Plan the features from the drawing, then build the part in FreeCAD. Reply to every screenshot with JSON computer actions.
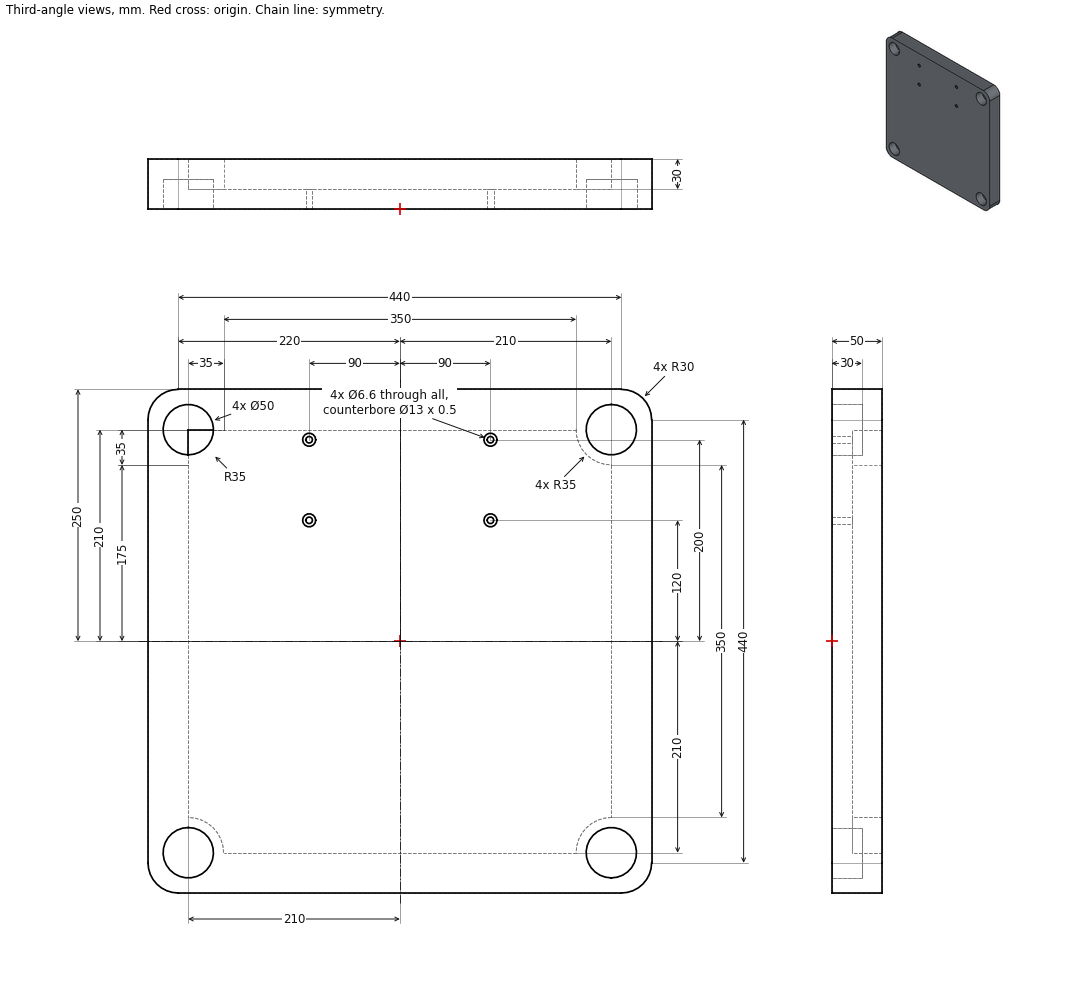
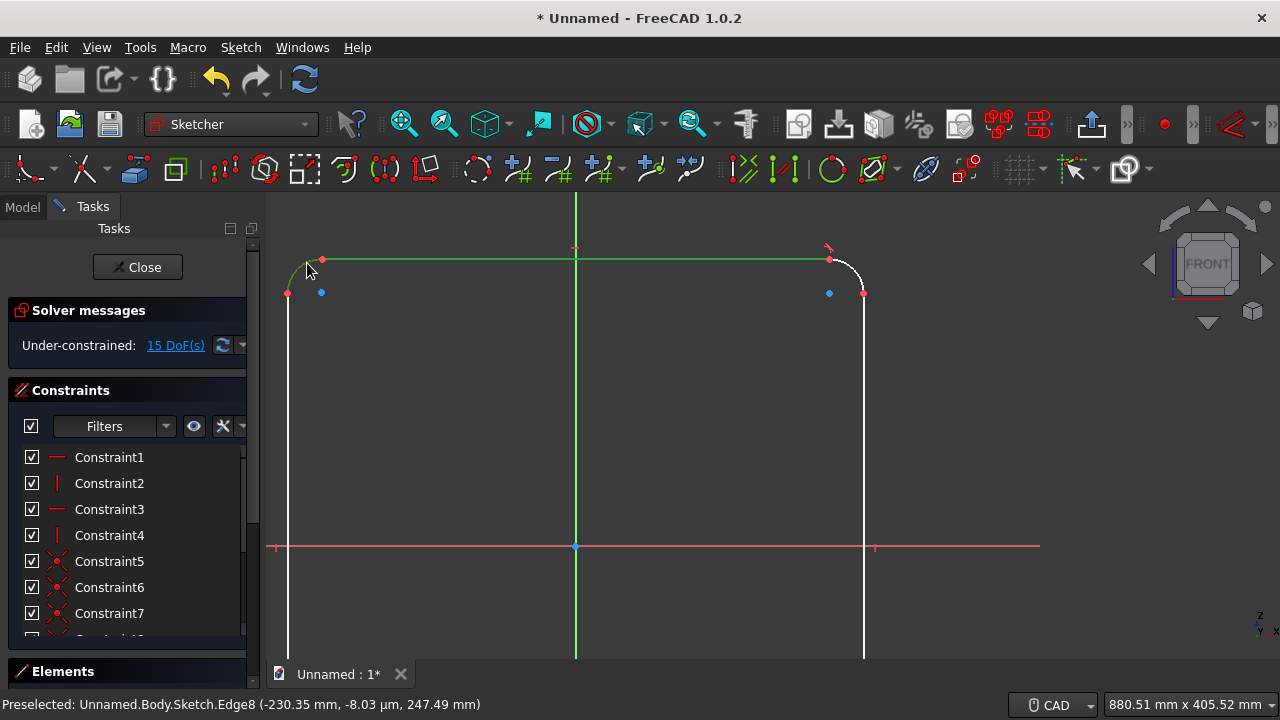
{"action": "key", "text": "t"}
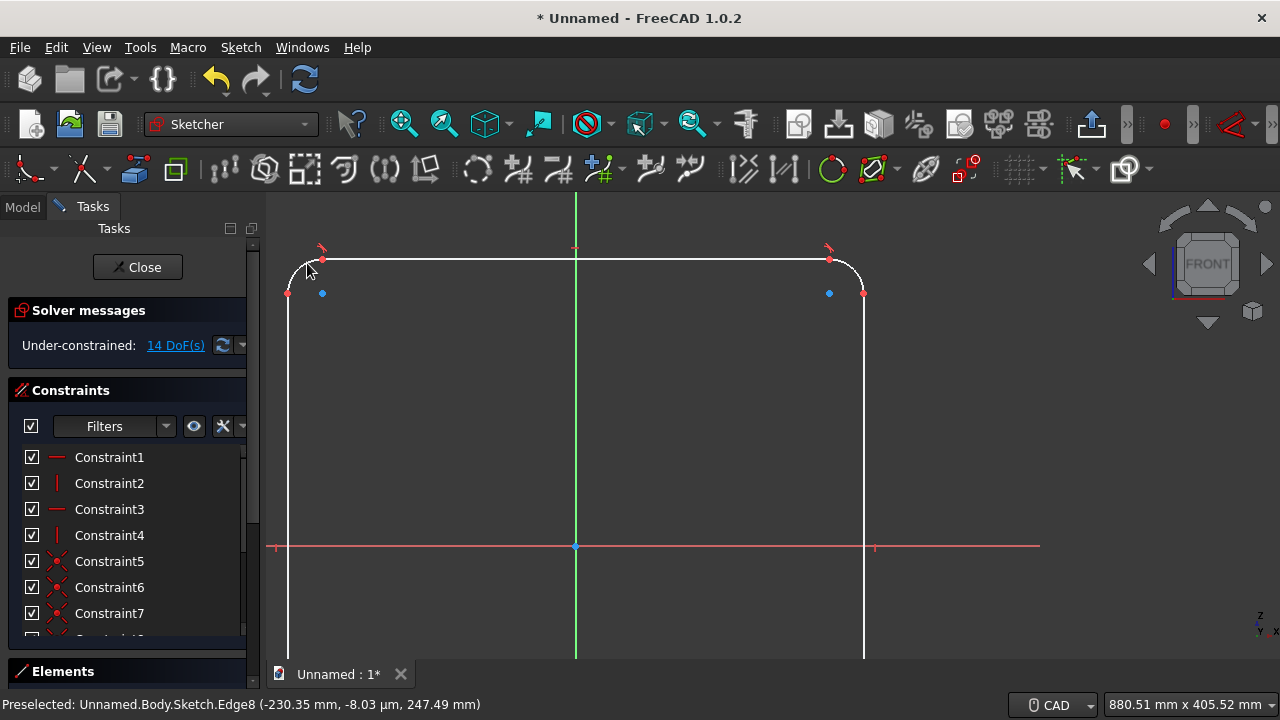
{"action": "left_click", "coordinate": [864, 446]}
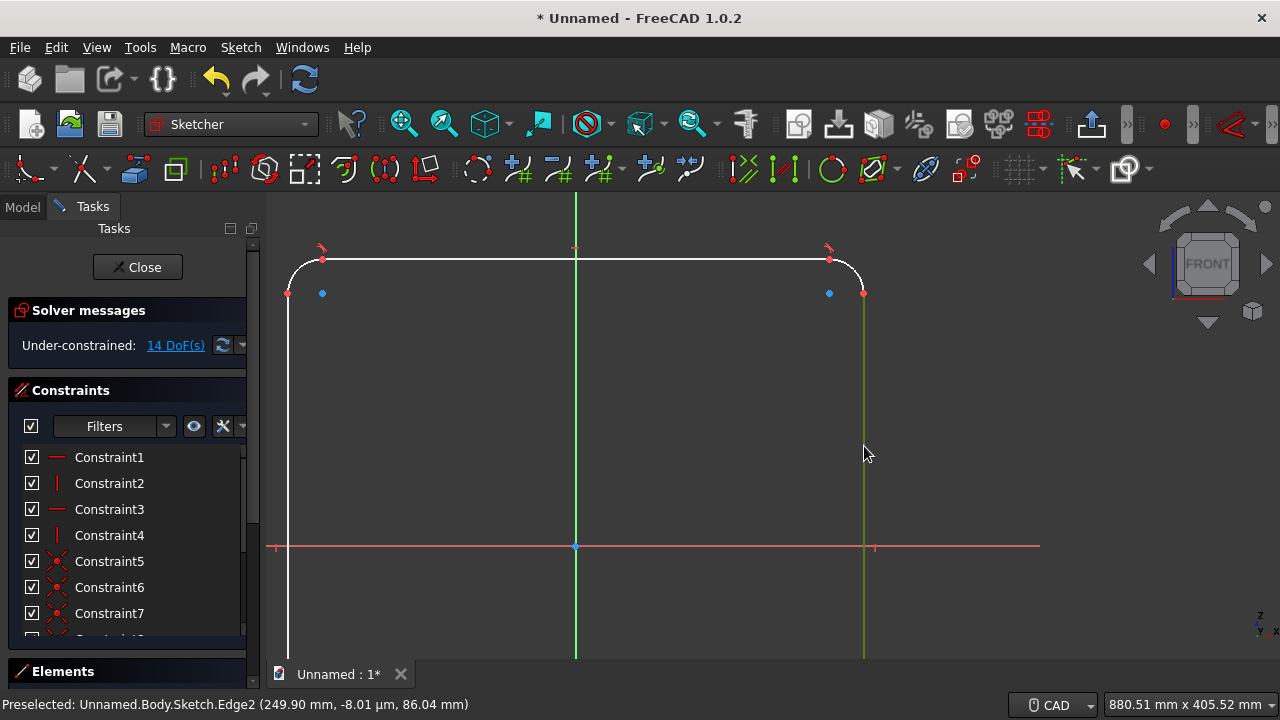
{"action": "left_click", "coordinate": [860, 278]}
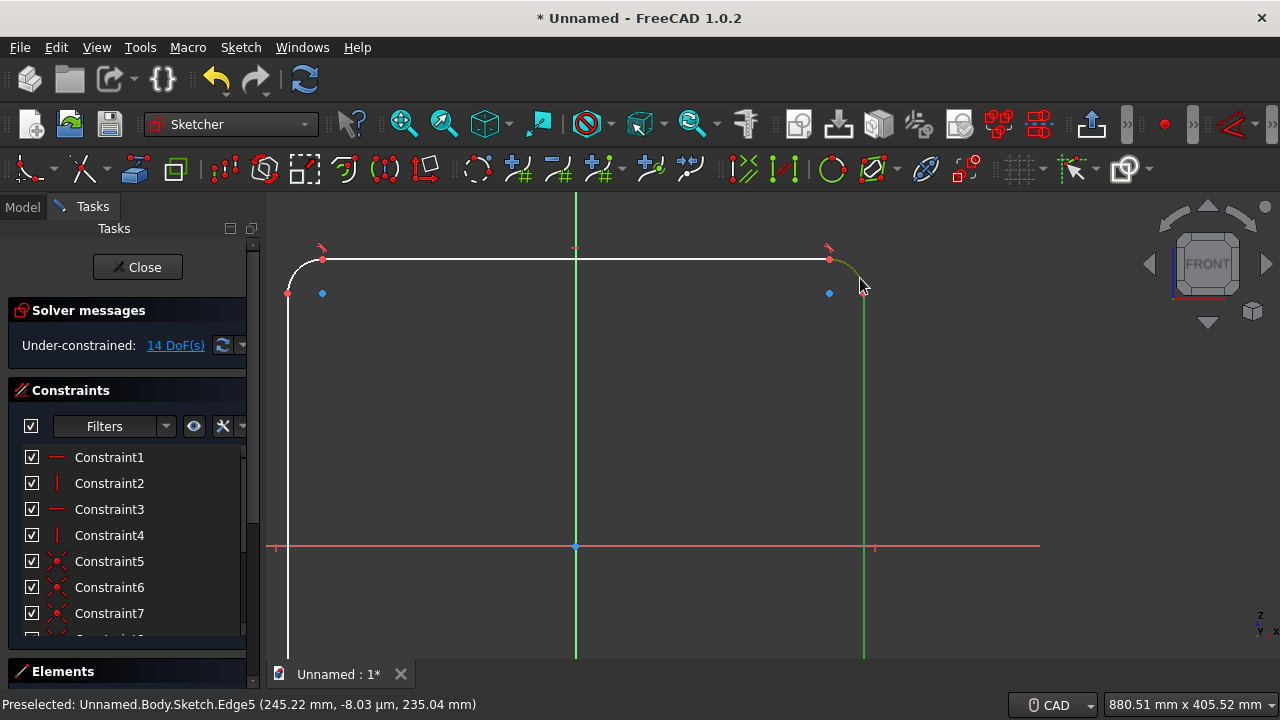
{"action": "key", "text": "t"}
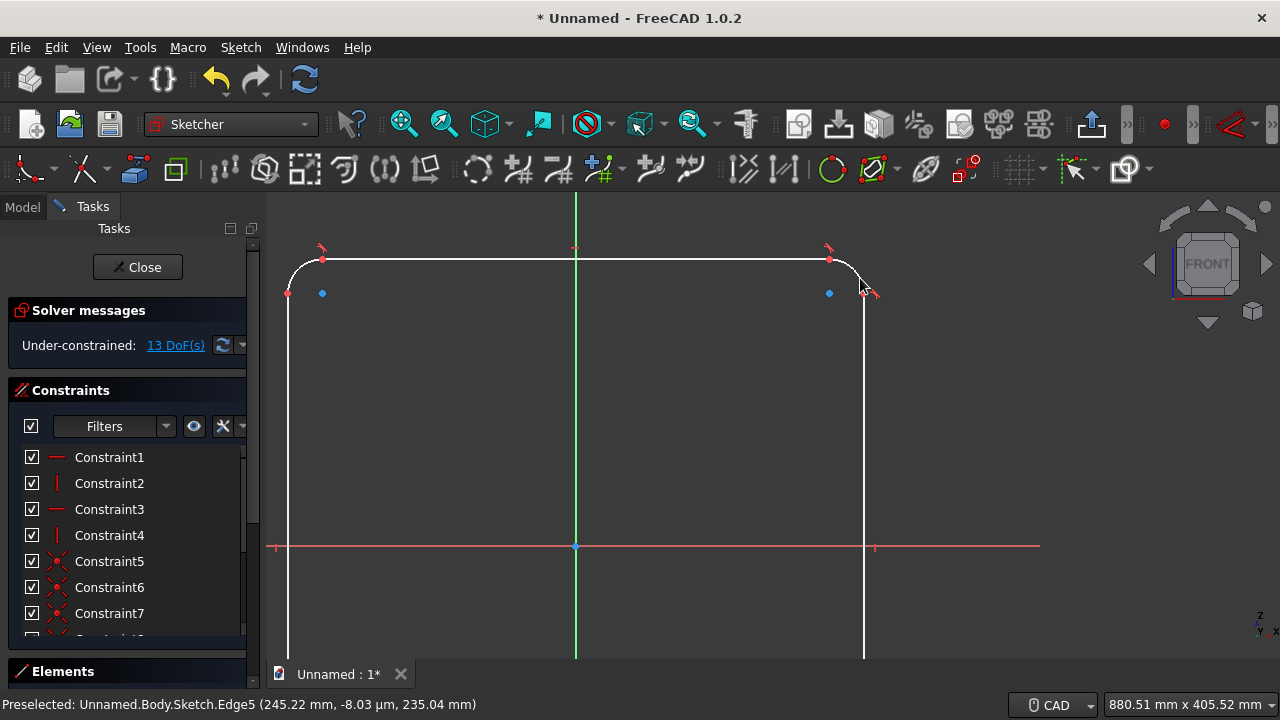
{"action": "left_click", "coordinate": [864, 446]}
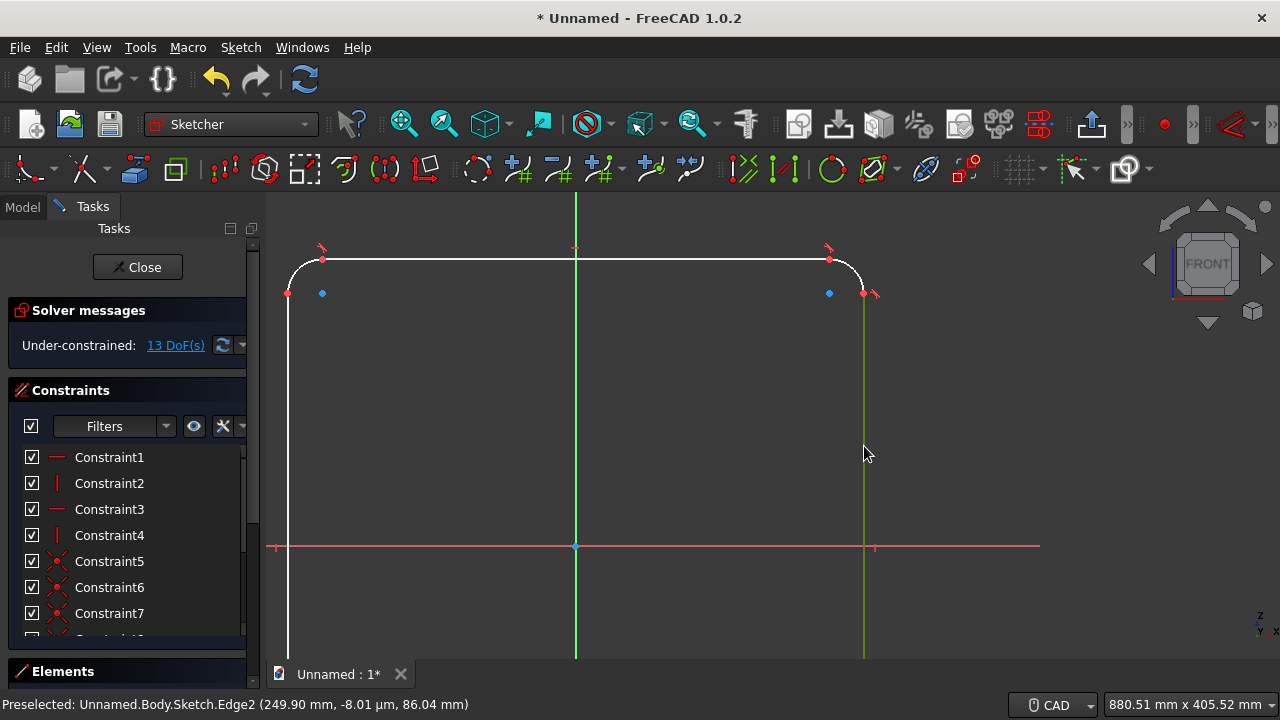
{"action": "scroll", "coordinate": [861, 279], "scroll_direction": "down", "scroll_amount": 3}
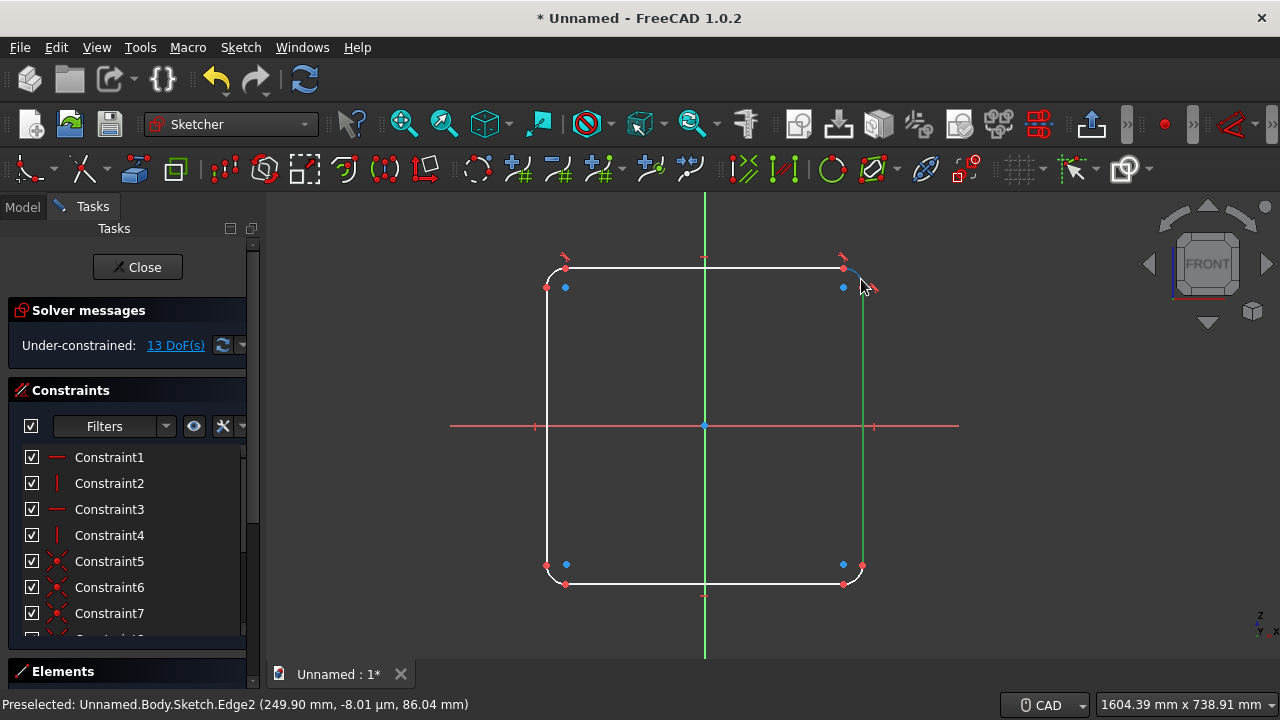
{"action": "scroll", "coordinate": [852, 582], "scroll_direction": "up", "scroll_amount": 3}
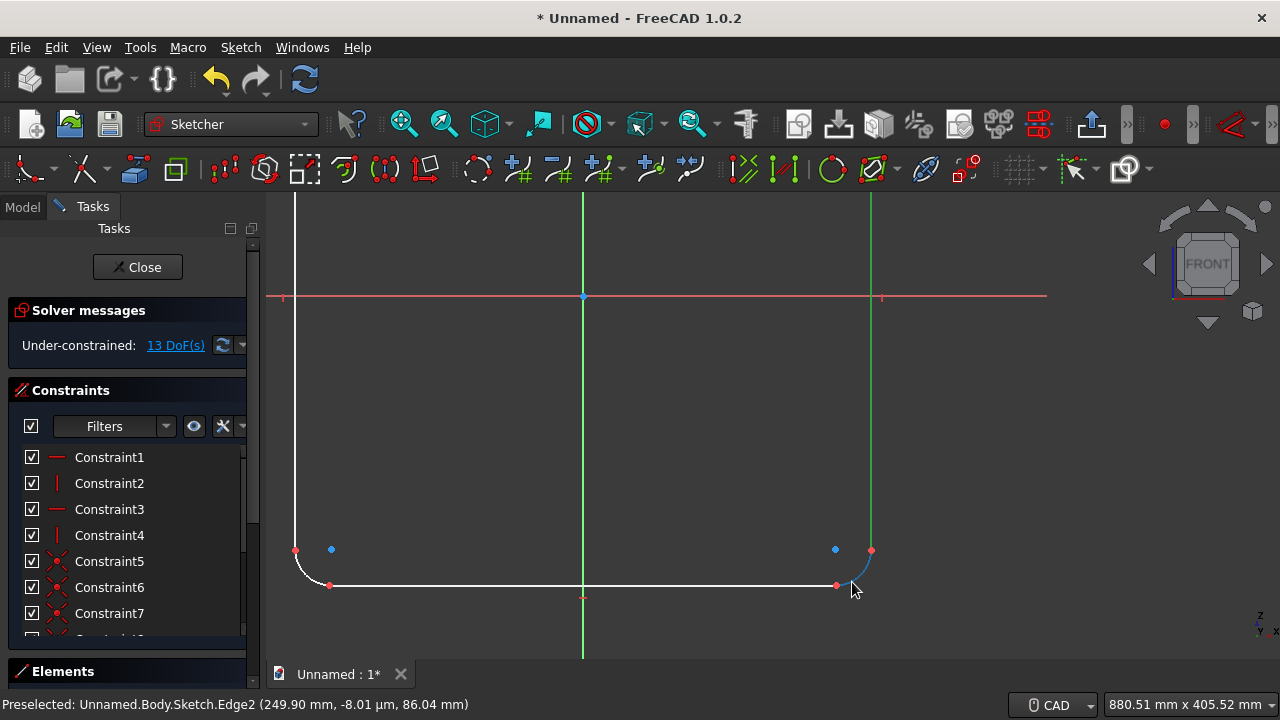
{"action": "left_click", "coordinate": [852, 581]}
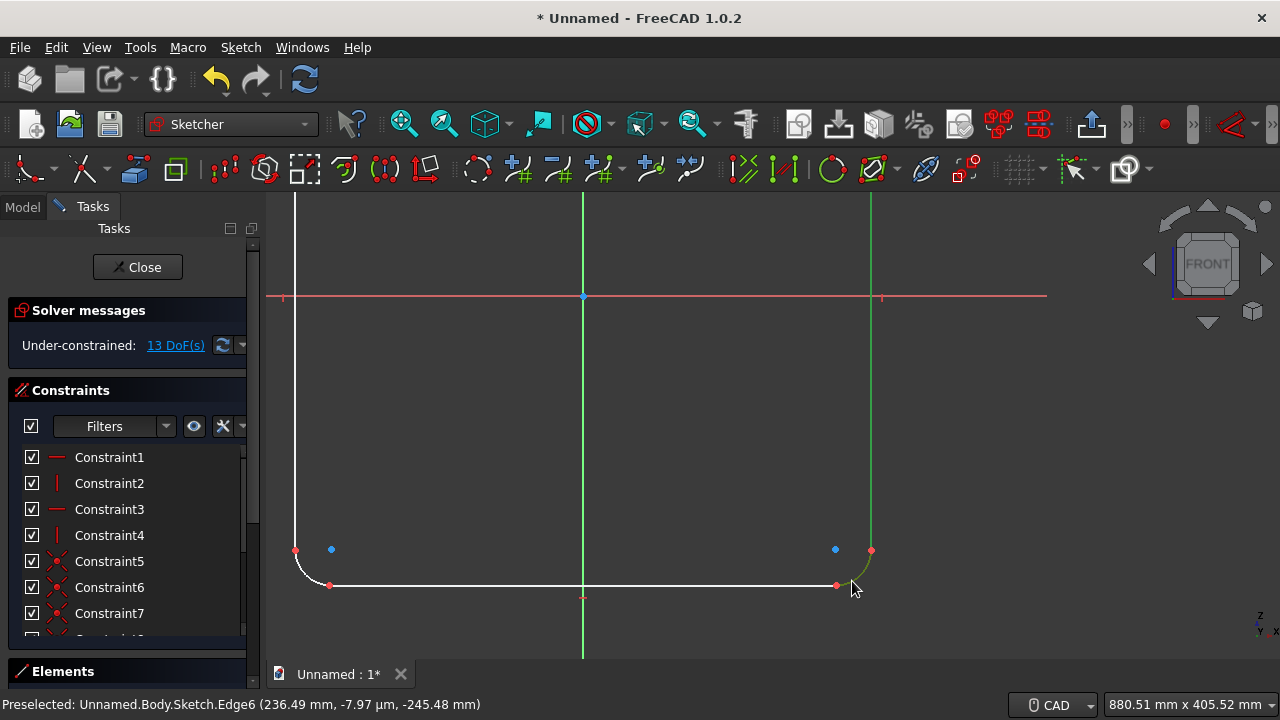
{"action": "key", "text": "t"}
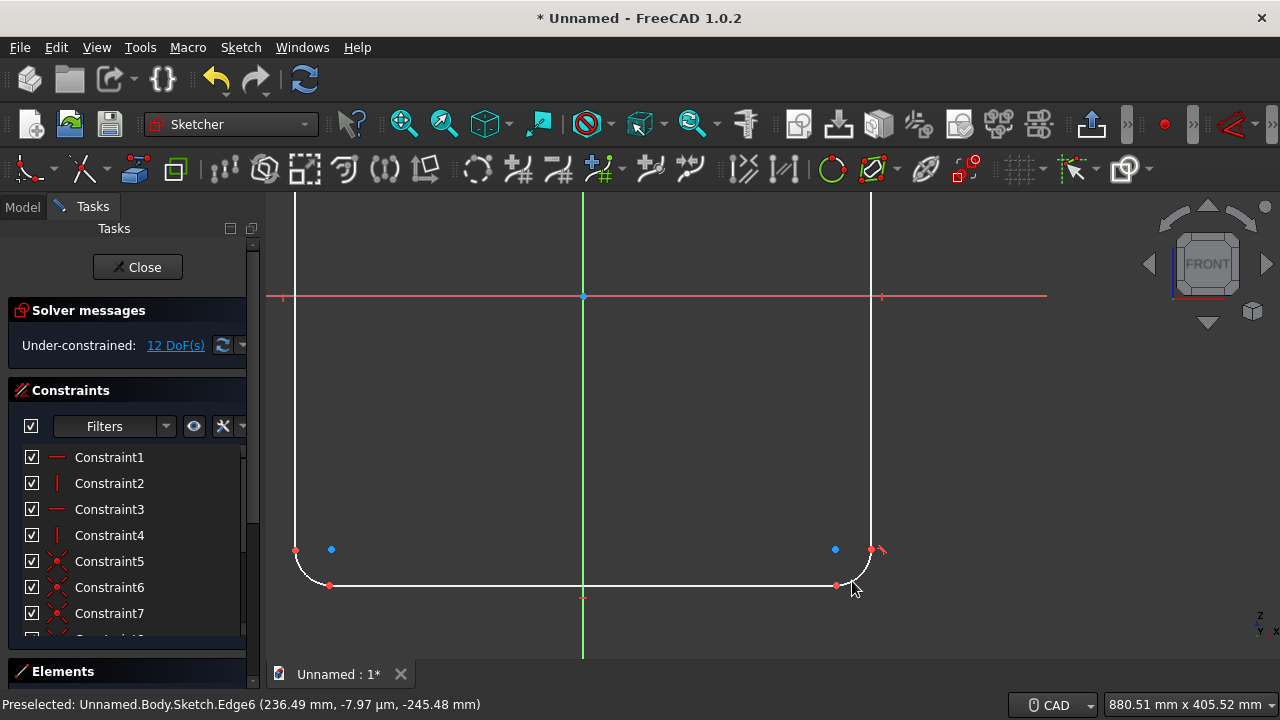
{"action": "left_click", "coordinate": [685, 586]}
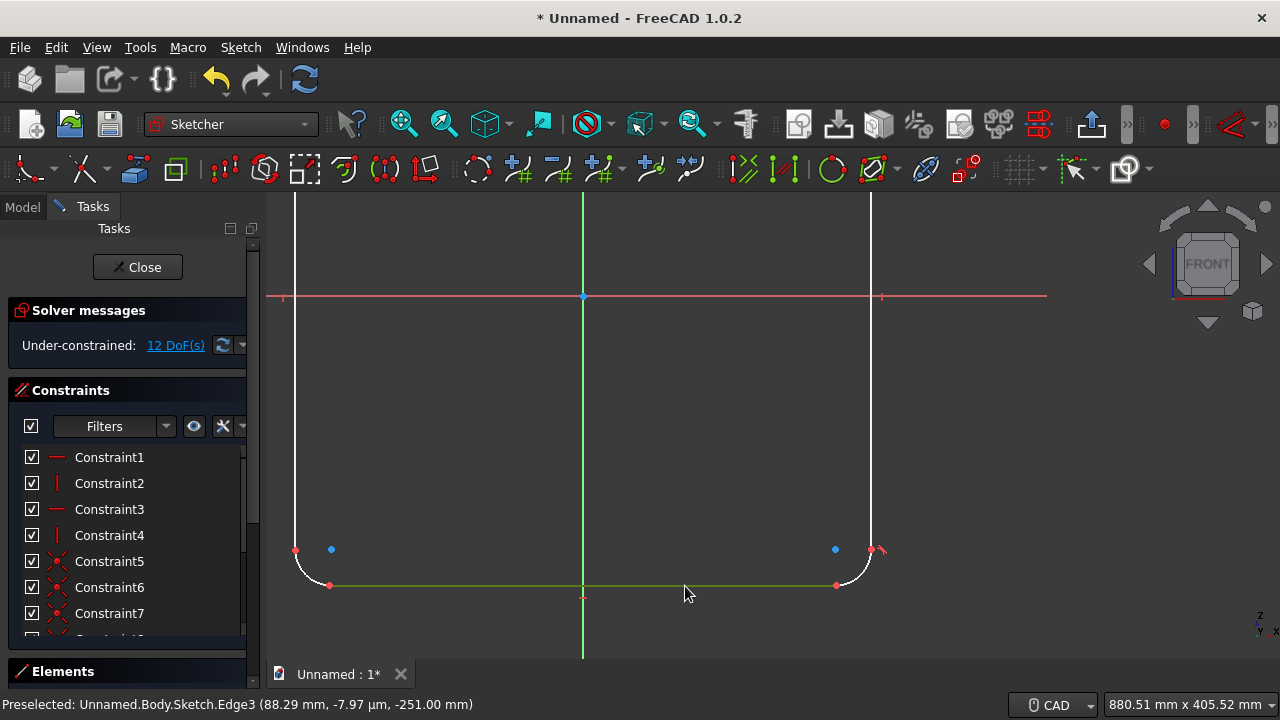
{"action": "left_click", "coordinate": [852, 581]}